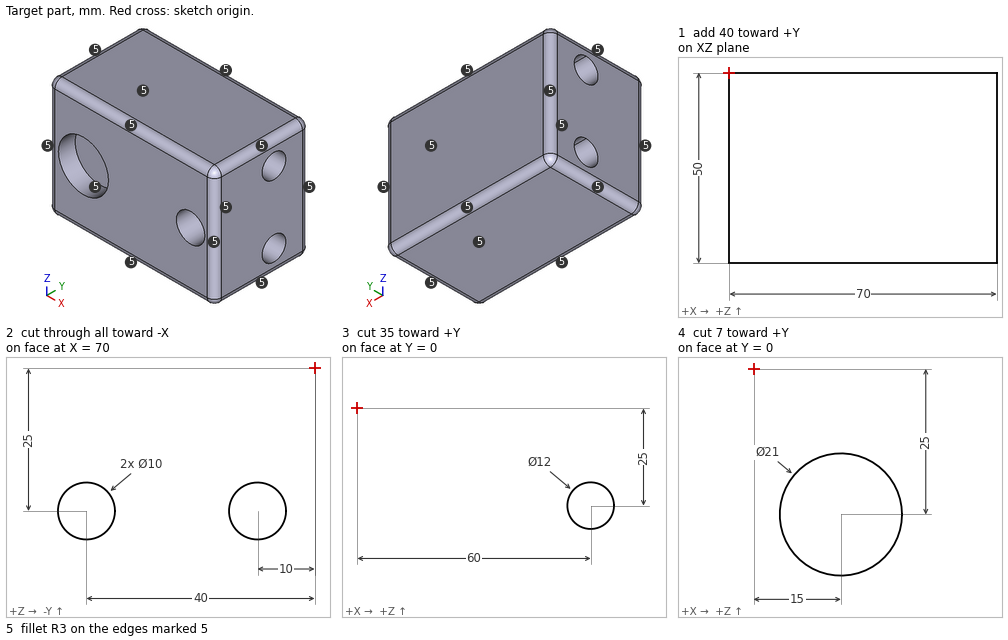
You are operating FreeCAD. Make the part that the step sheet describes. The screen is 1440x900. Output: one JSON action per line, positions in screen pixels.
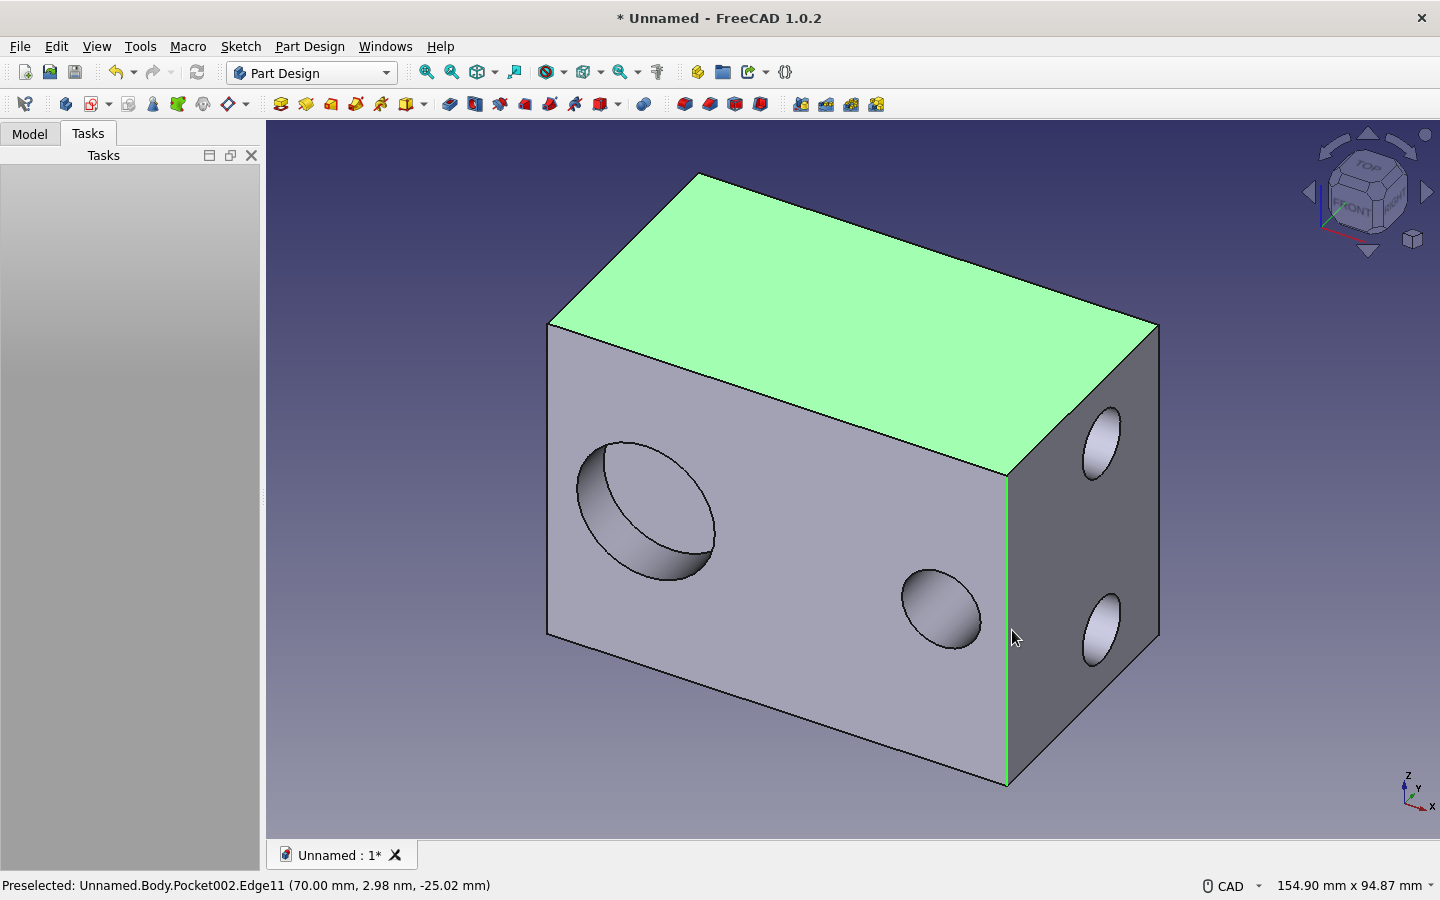
{"action": "key", "text": "0"}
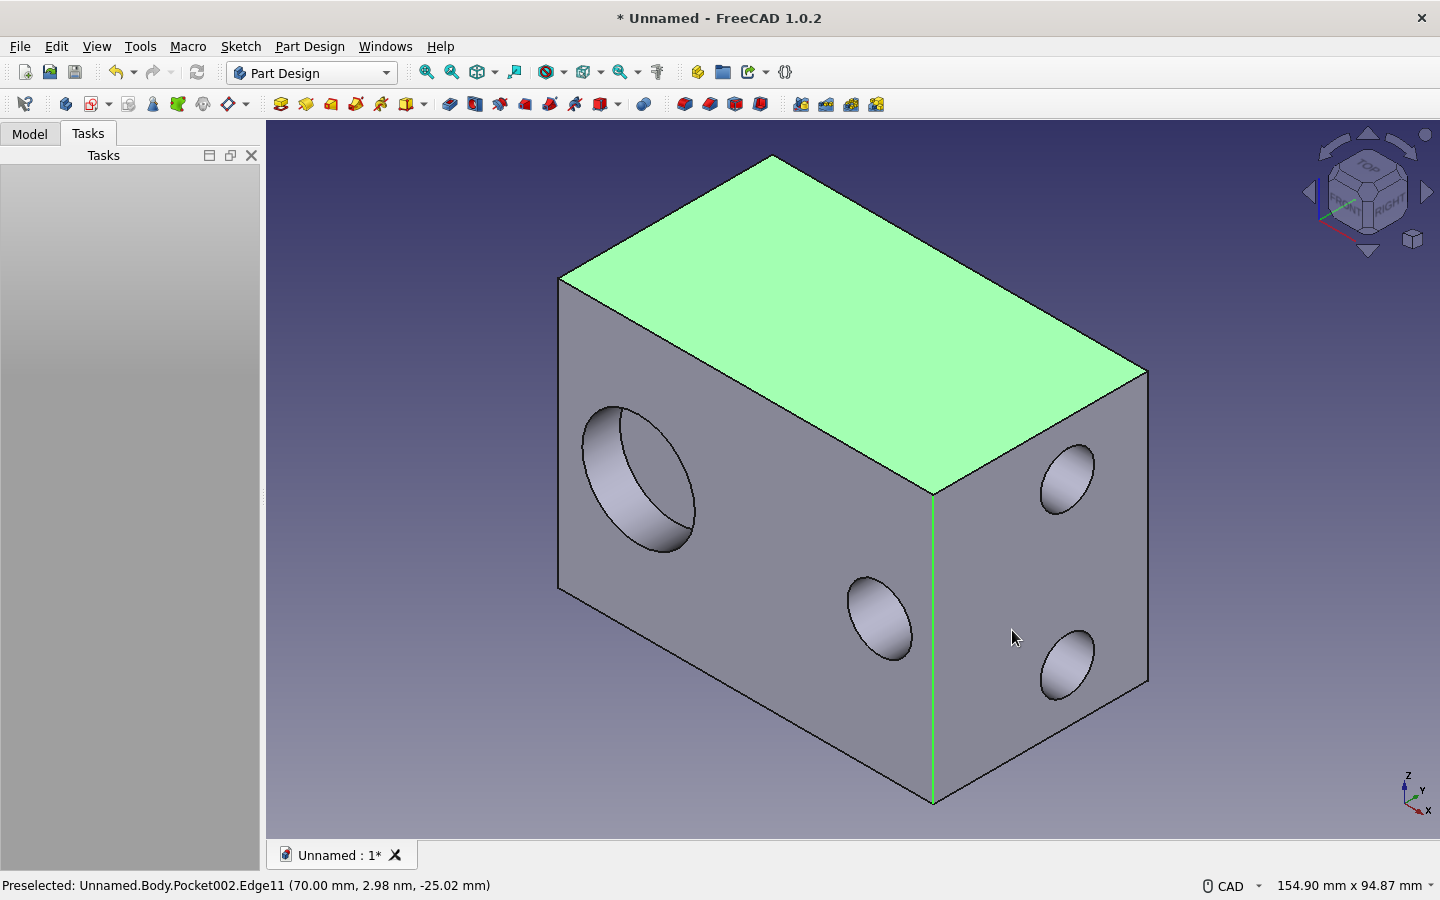
{"action": "key", "text": "2"}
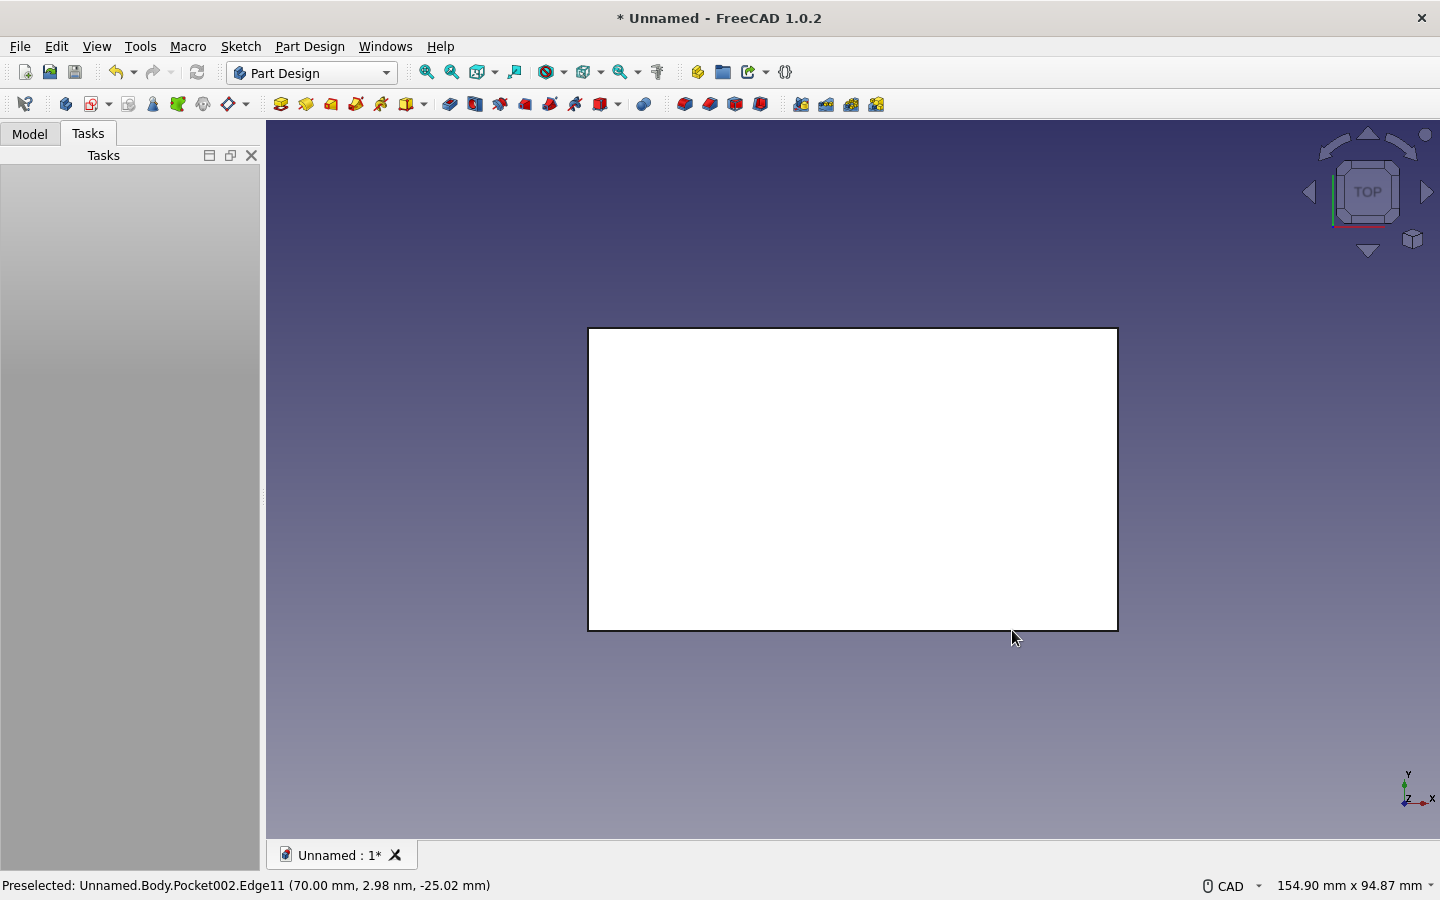
{"action": "key", "text": "1"}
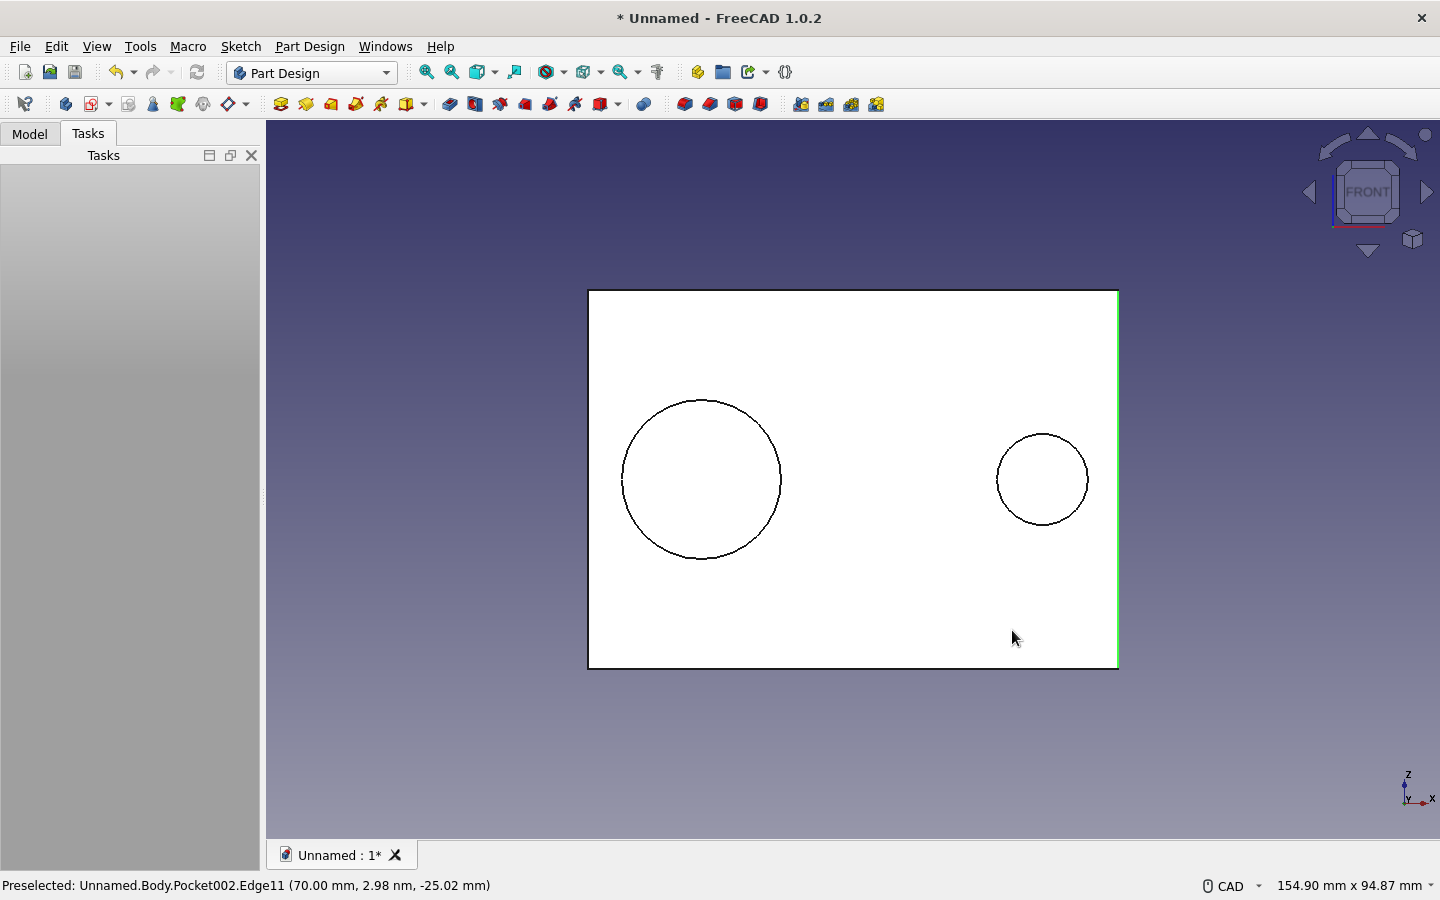
{"action": "key", "text": "3"}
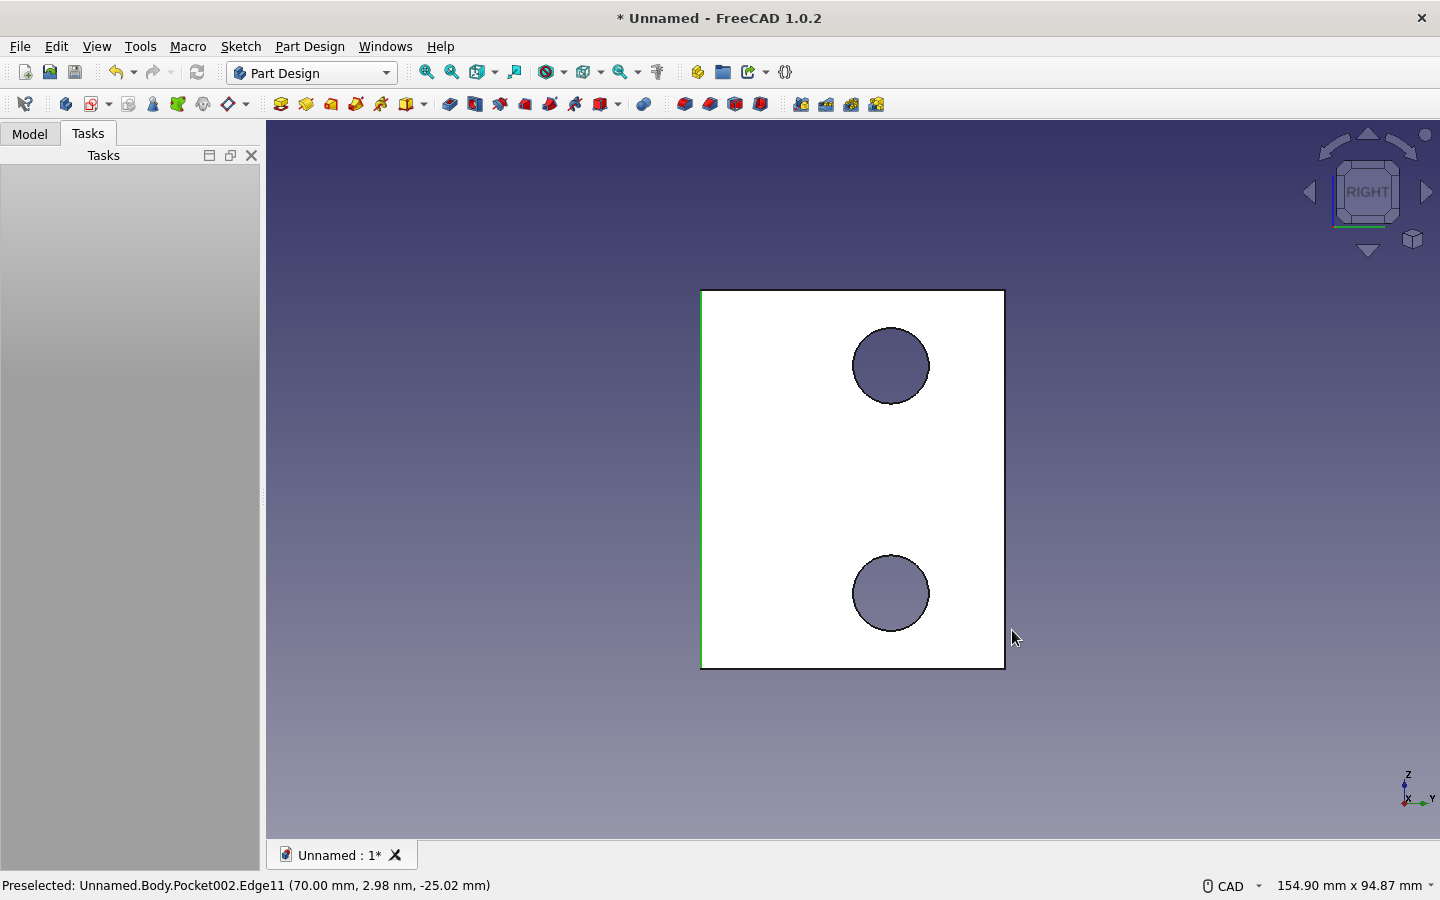
{"action": "key", "text": "5"}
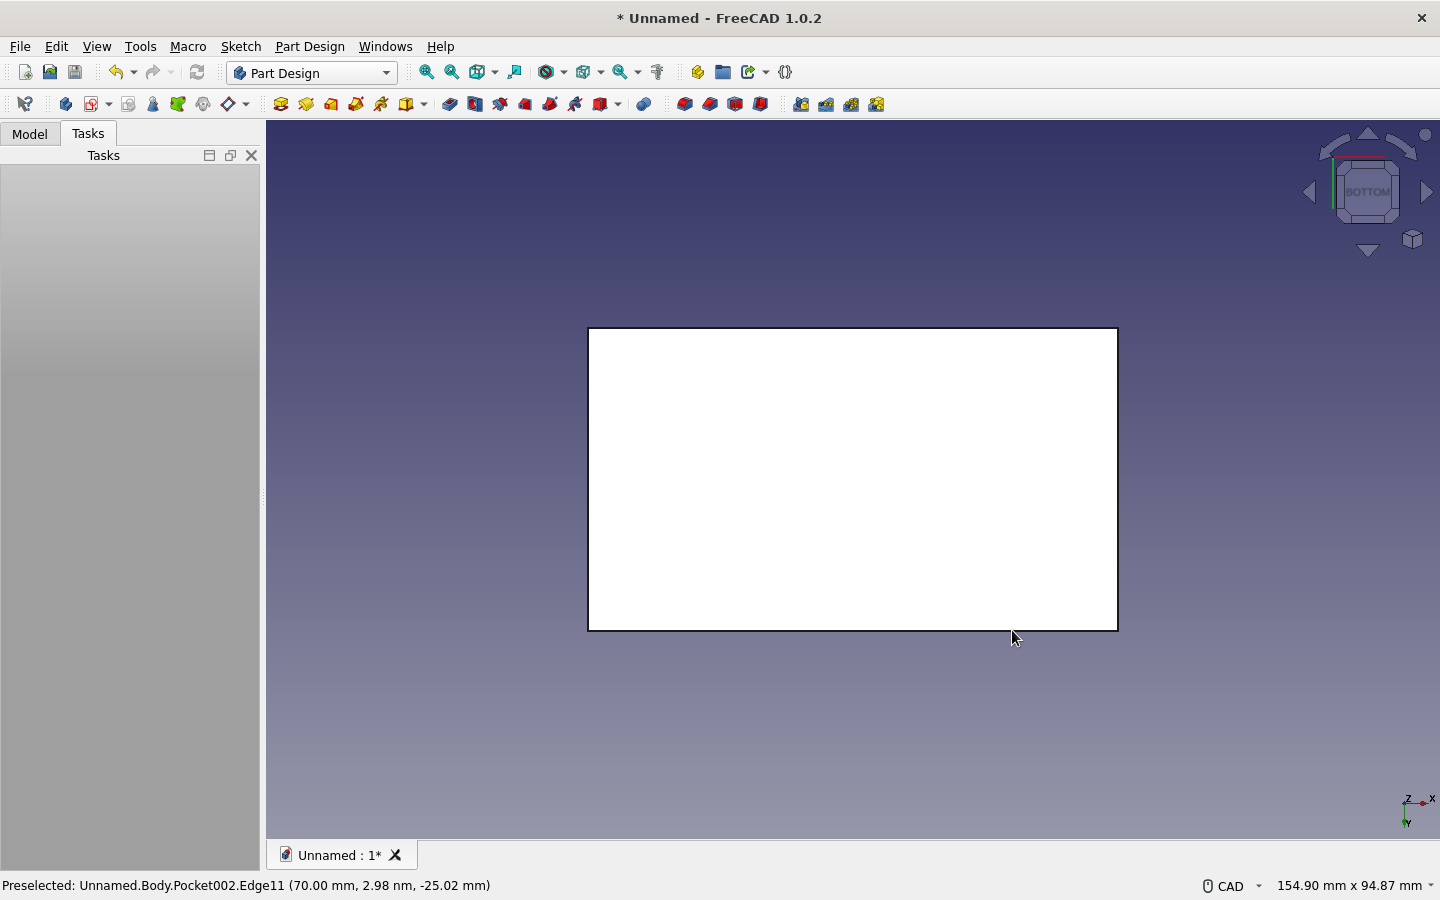
{"action": "left_click", "coordinate": [929, 478], "text": "ctrl"}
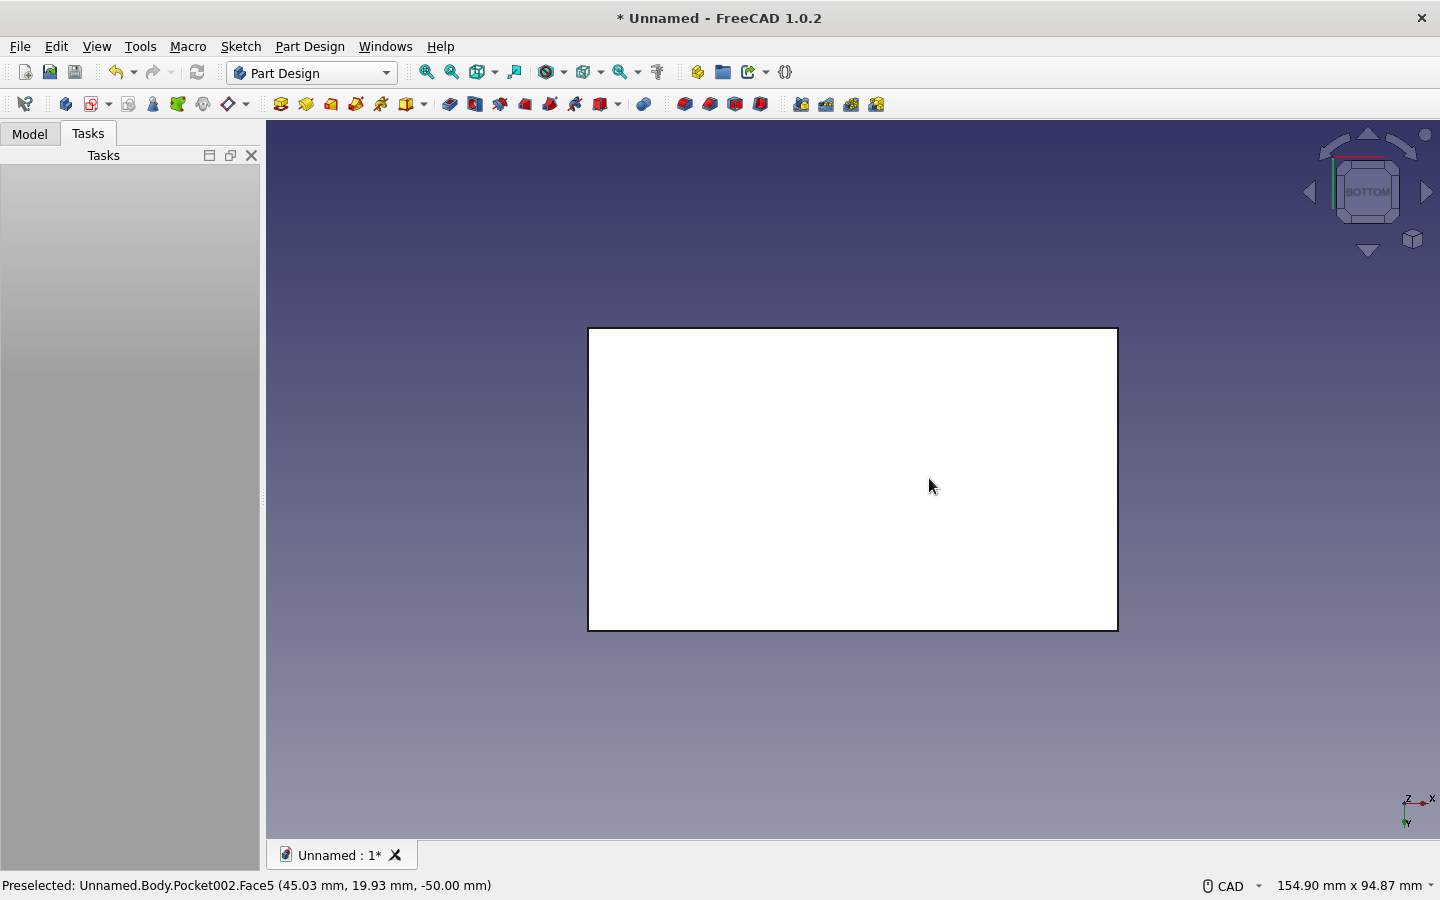
{"action": "key", "text": "4"}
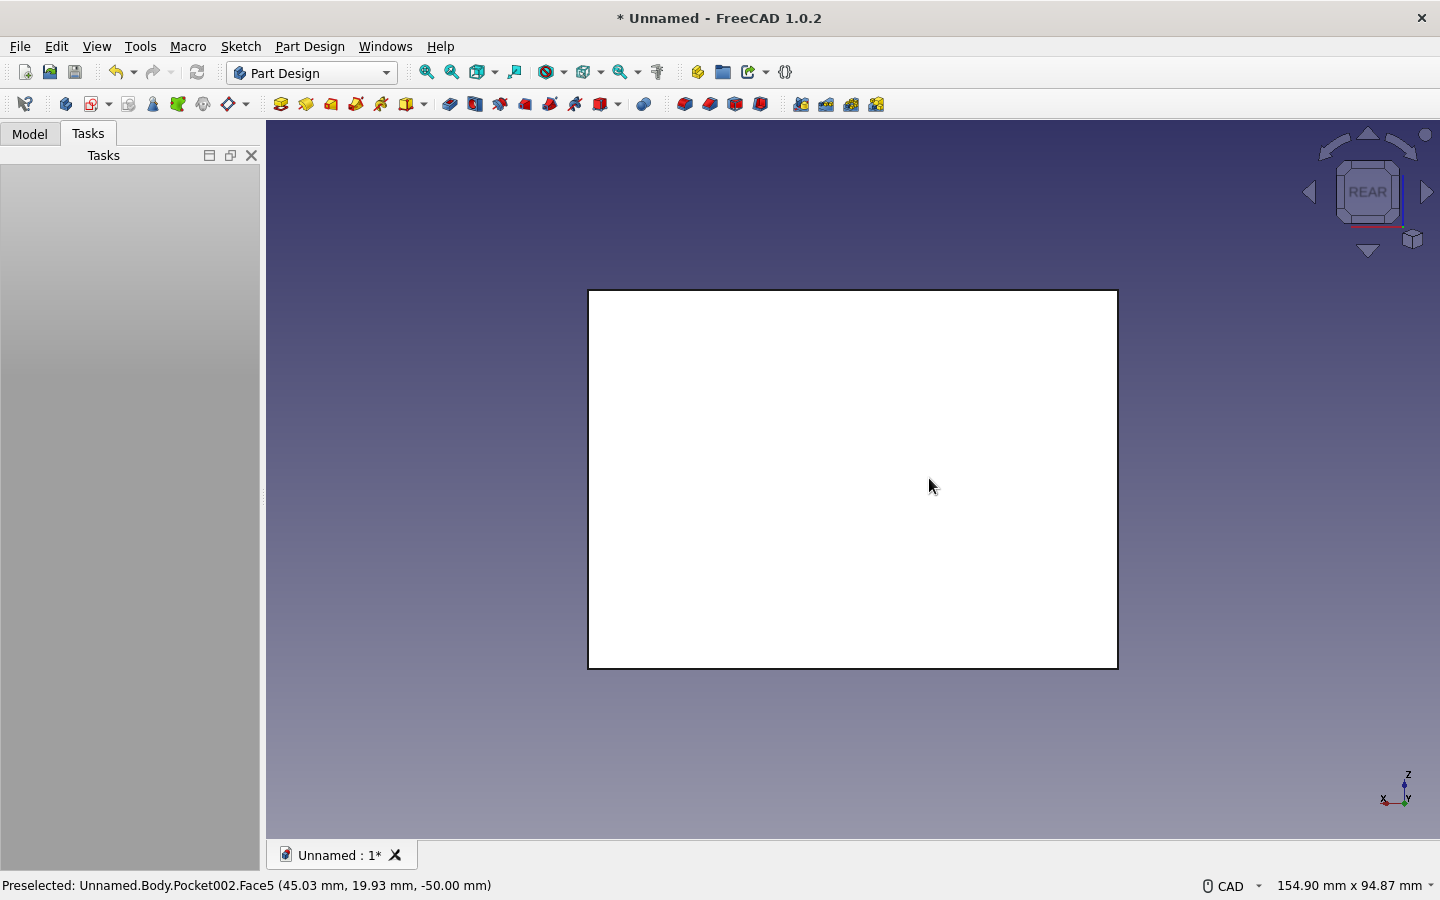
{"action": "left_click", "coordinate": [853, 478], "text": "ctrl"}